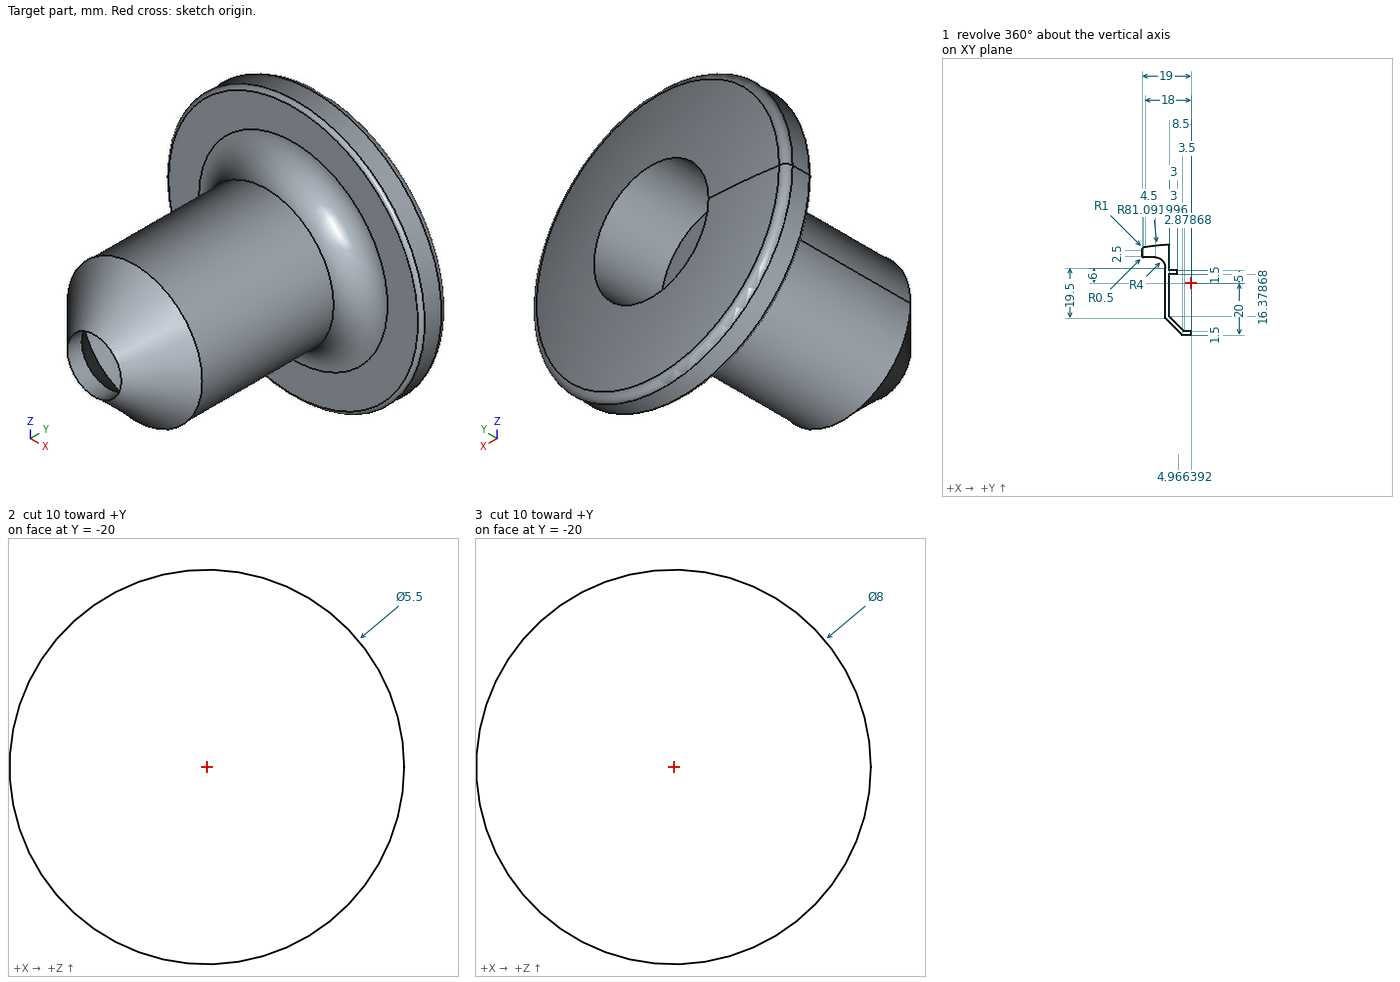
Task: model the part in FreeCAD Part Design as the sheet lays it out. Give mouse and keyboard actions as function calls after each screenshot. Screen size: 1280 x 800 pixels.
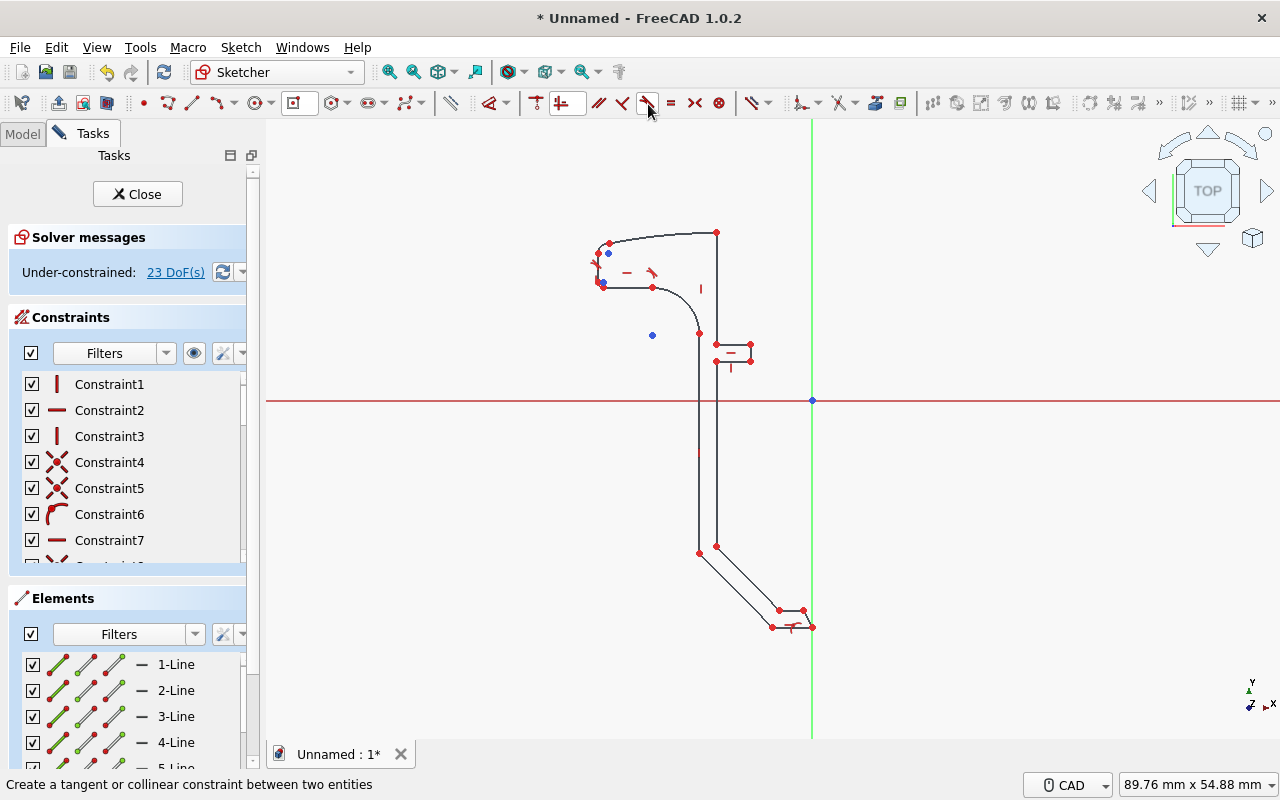
click(699, 399)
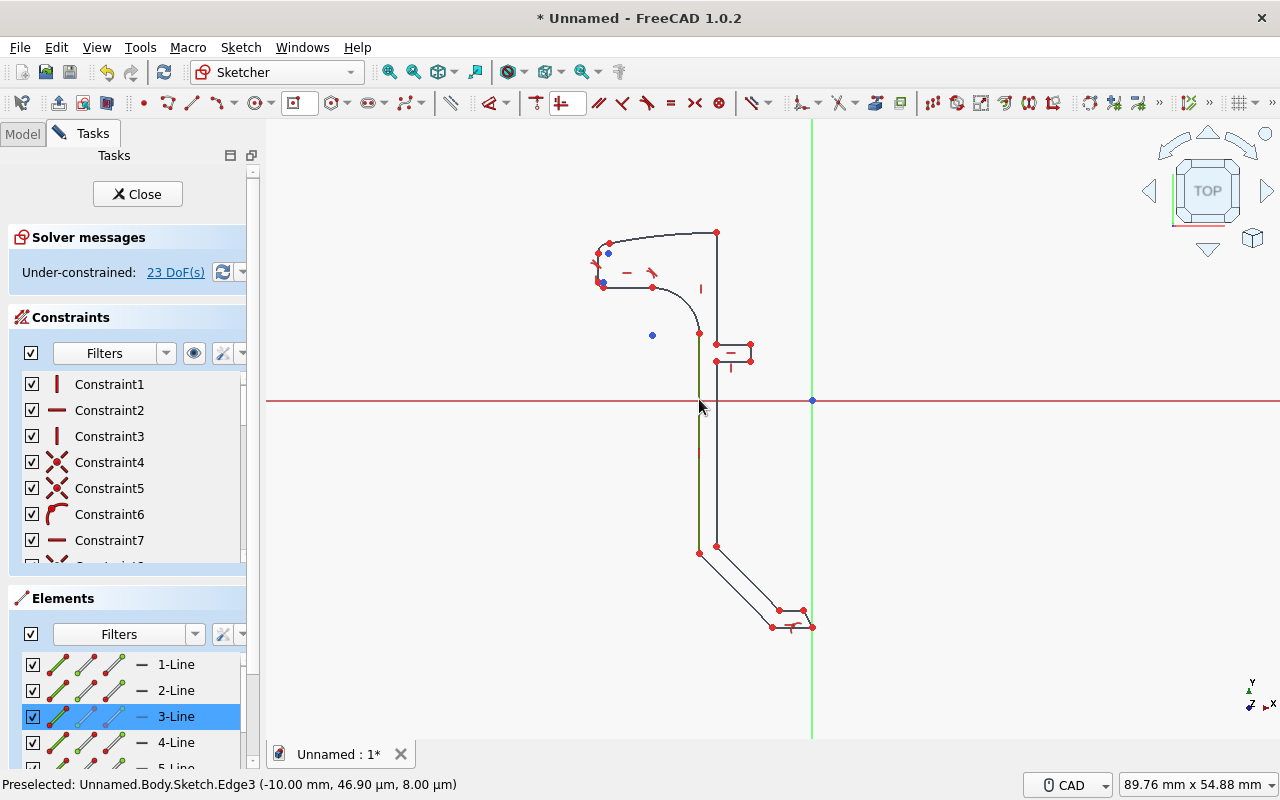
click(694, 313)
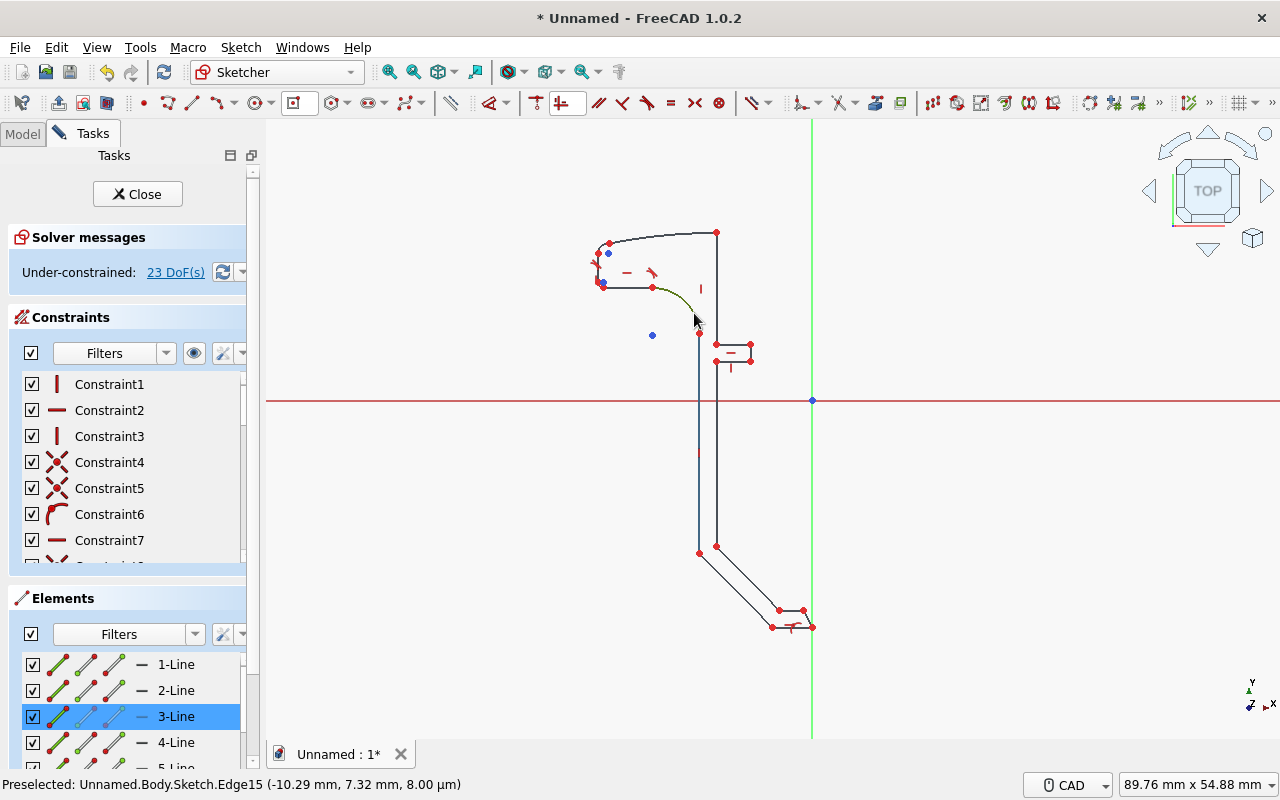
click(648, 104)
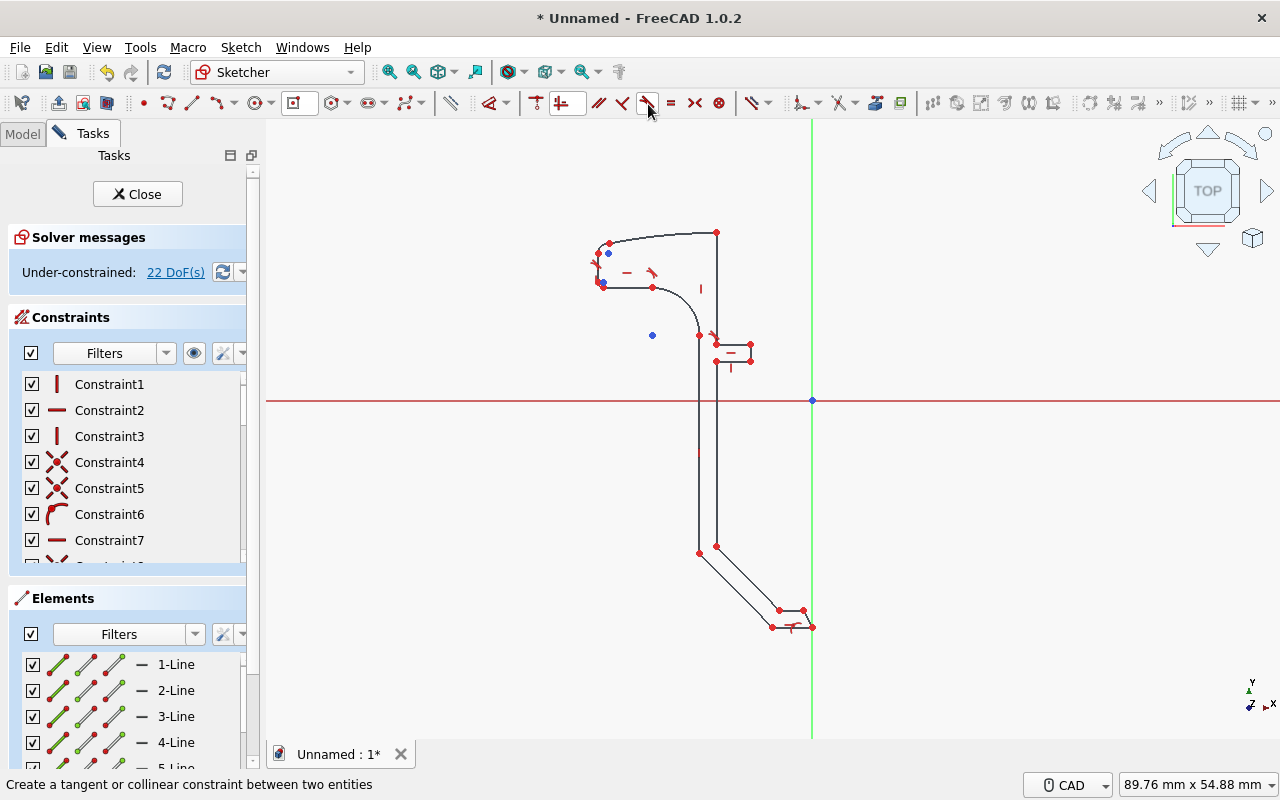
scroll(809, 621, up, 4)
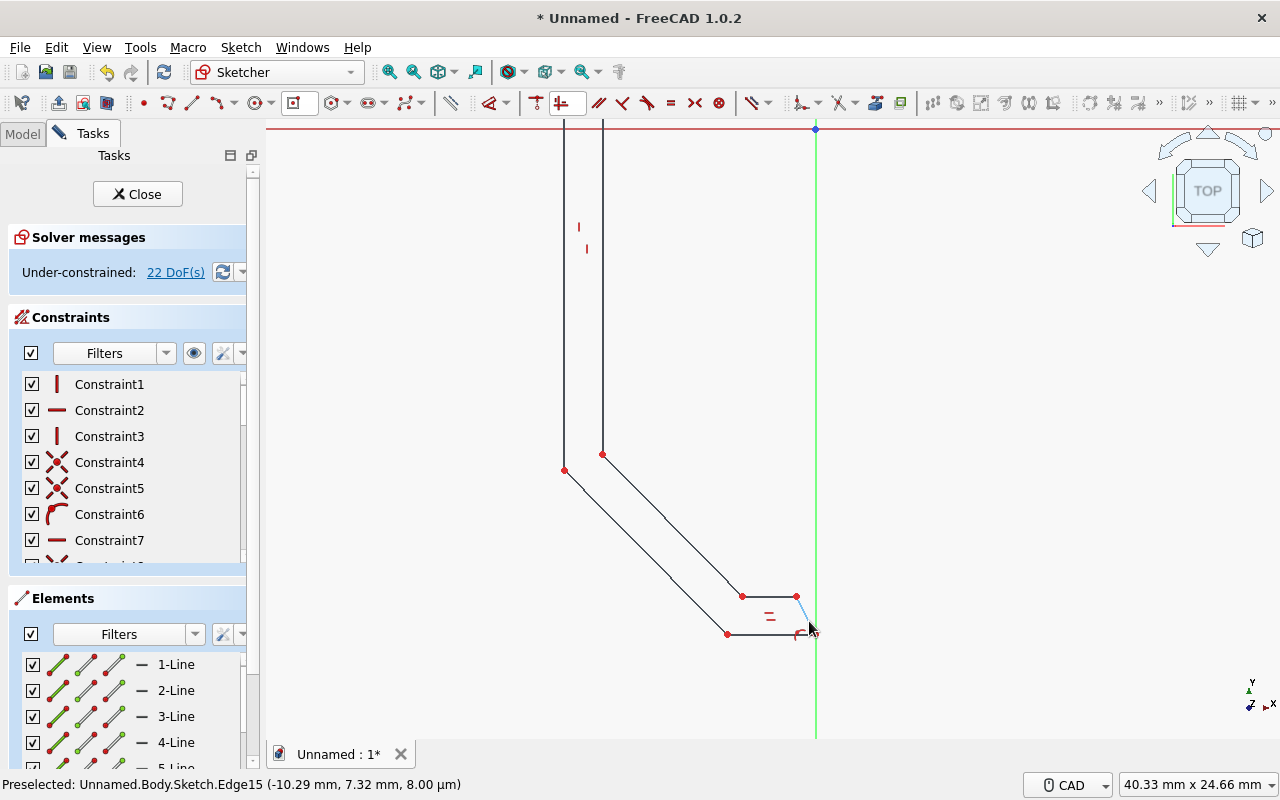
click(808, 620)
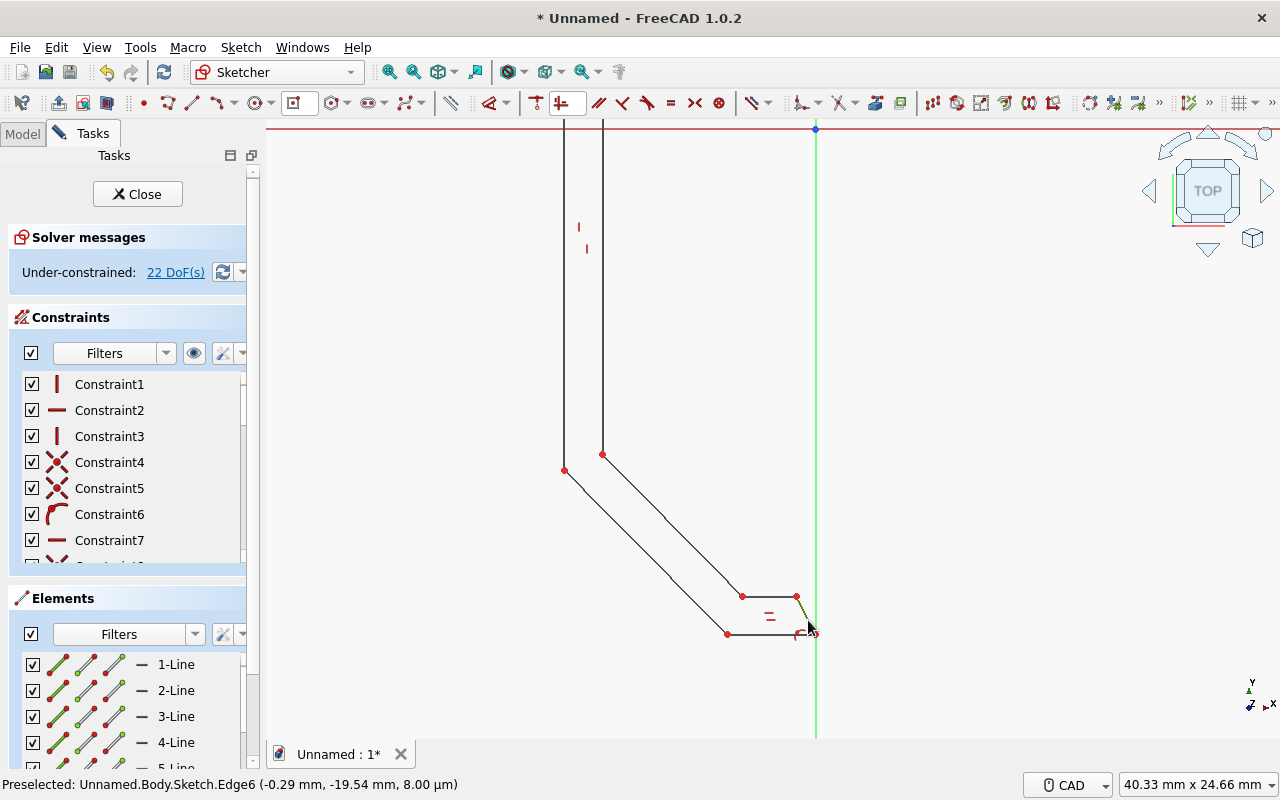
click(580, 104)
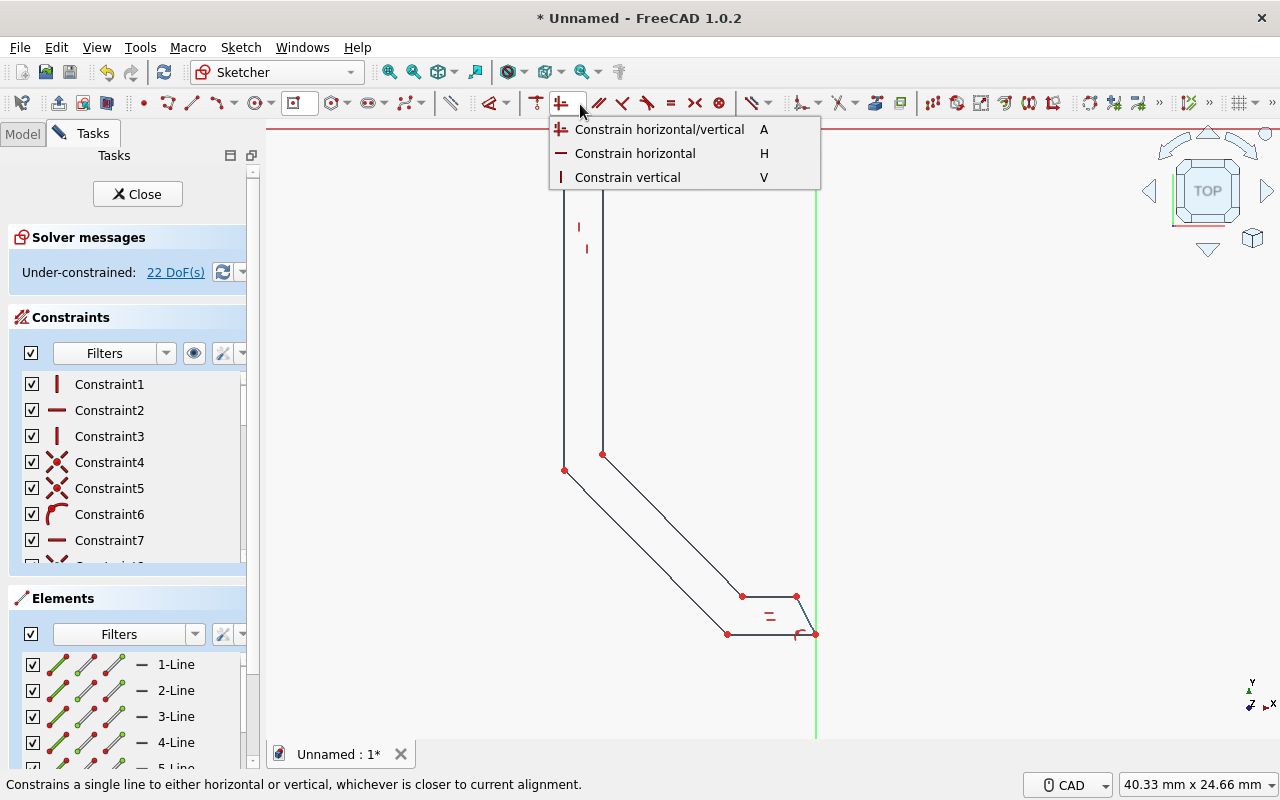
click(685, 177)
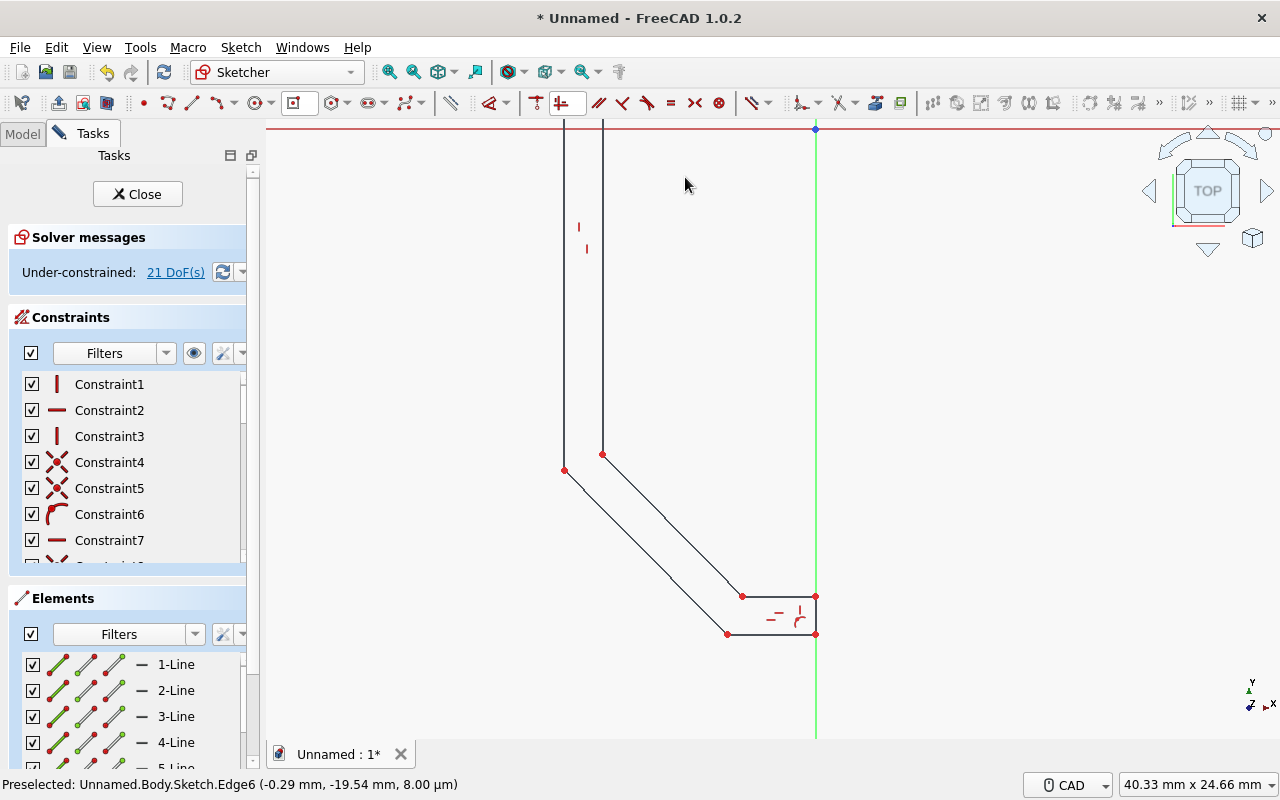
click(490, 104)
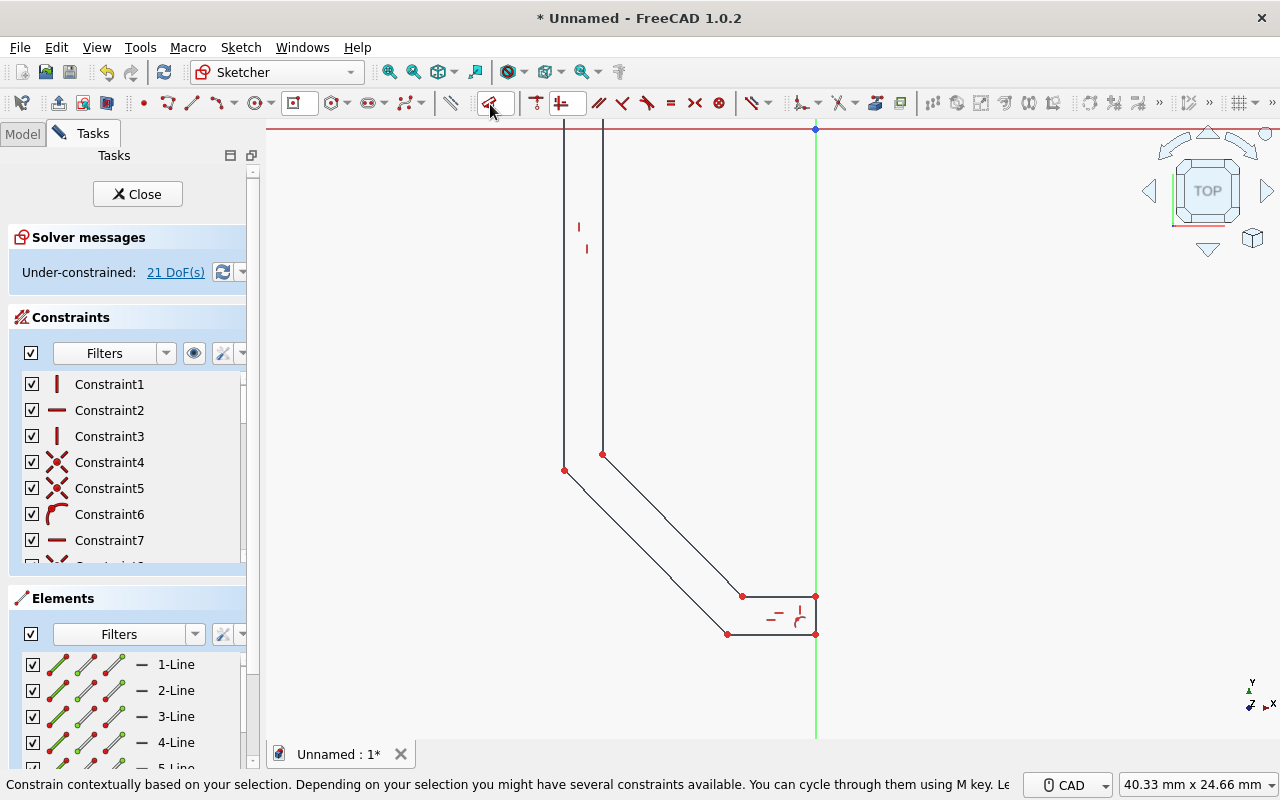
scroll(809, 622, down, 4)